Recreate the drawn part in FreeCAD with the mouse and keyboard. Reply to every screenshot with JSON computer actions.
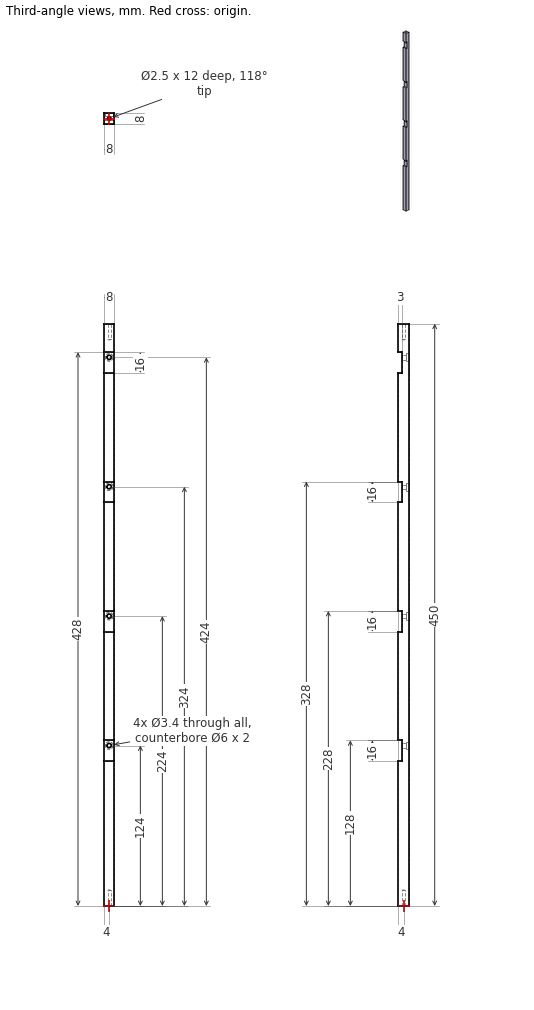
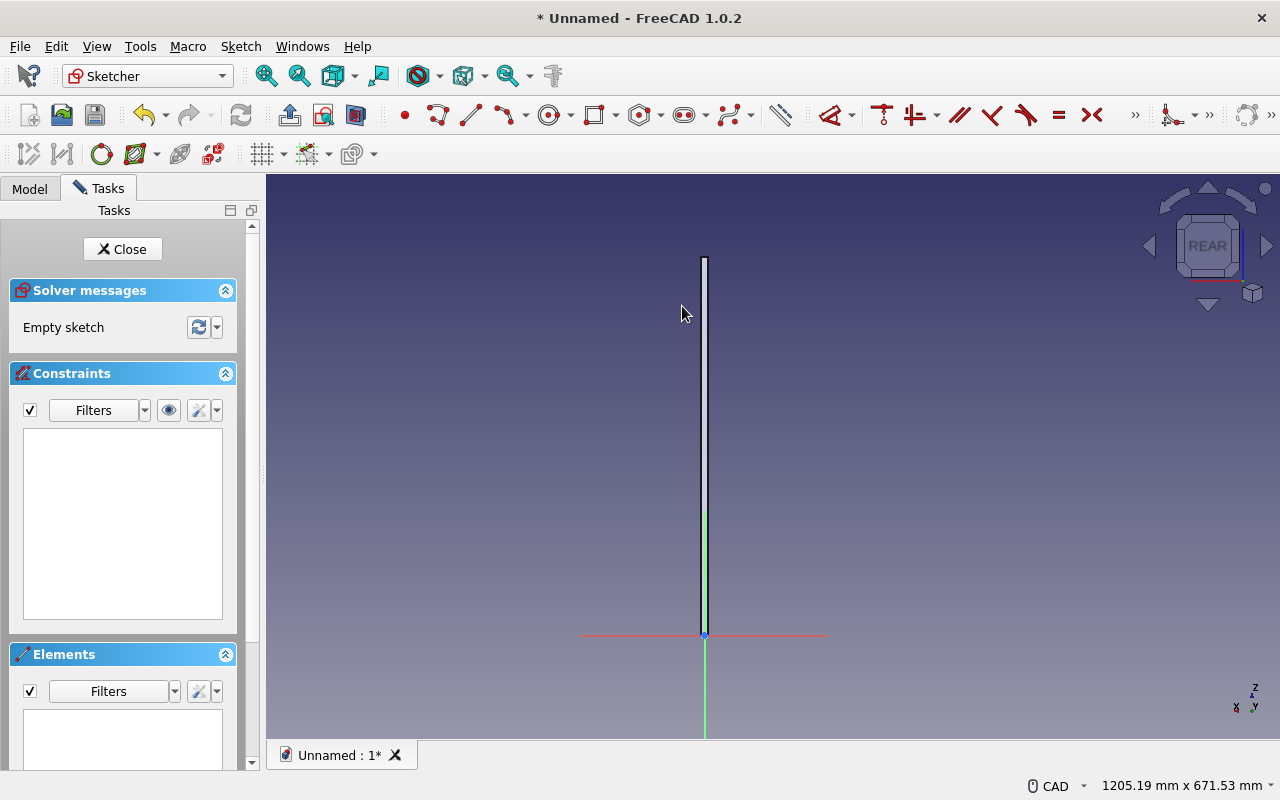
{"action": "key", "text": "g c"}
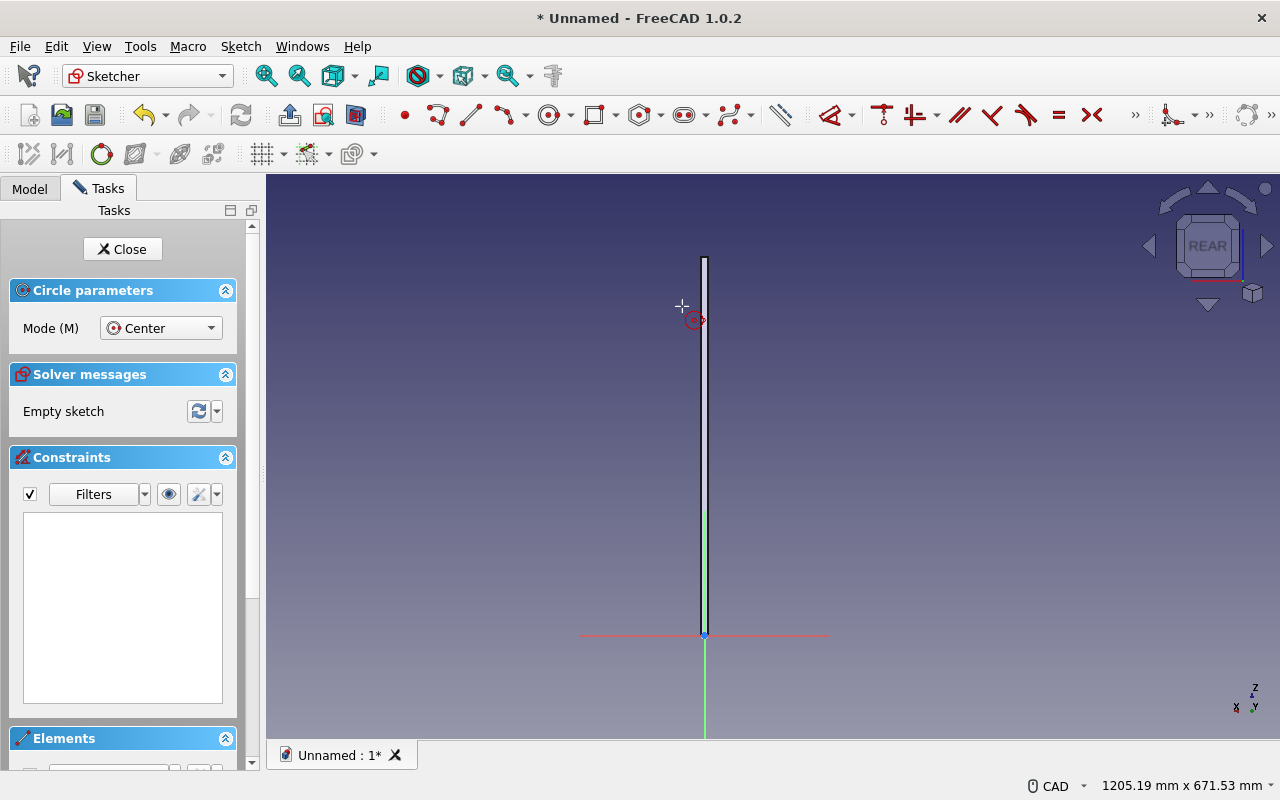
{"action": "scroll", "coordinate": [705, 531], "scroll_direction": "up", "scroll_amount": 14}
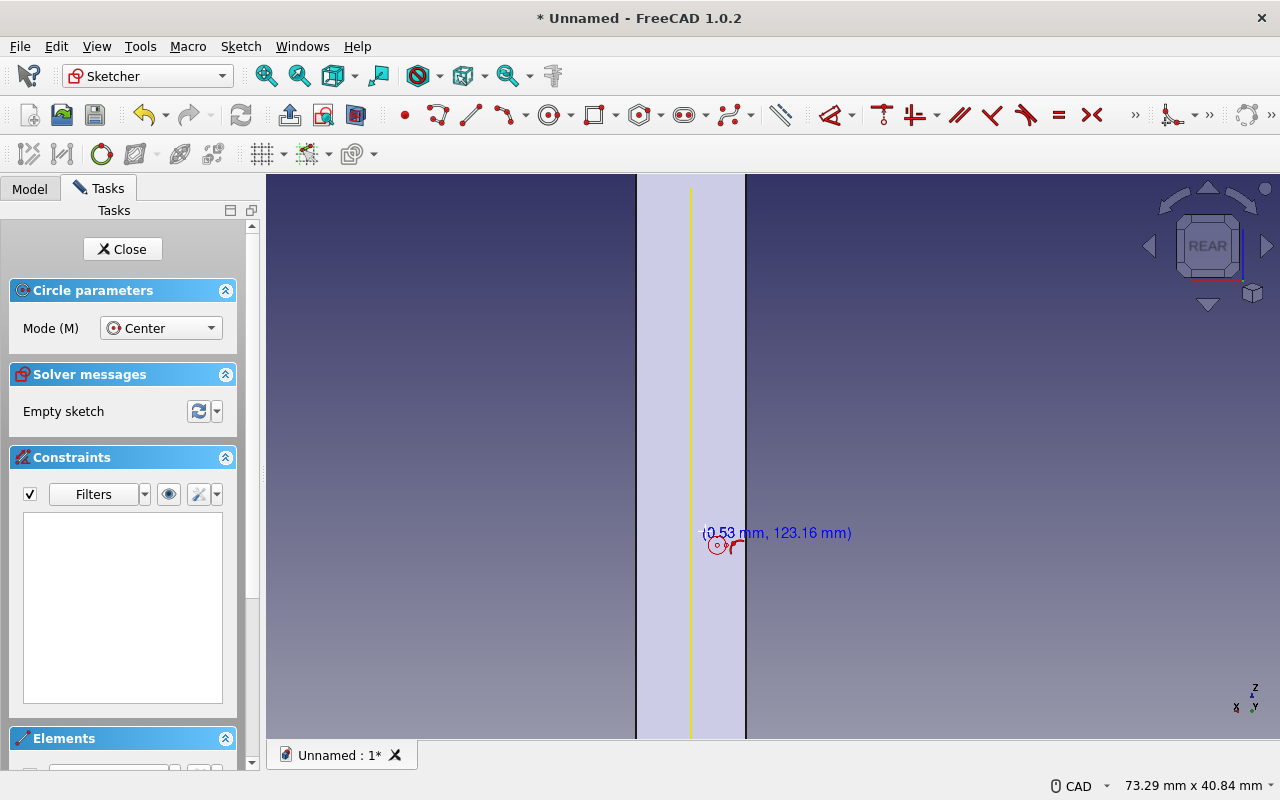
{"action": "scroll", "coordinate": [705, 532], "scroll_direction": "down", "scroll_amount": 14}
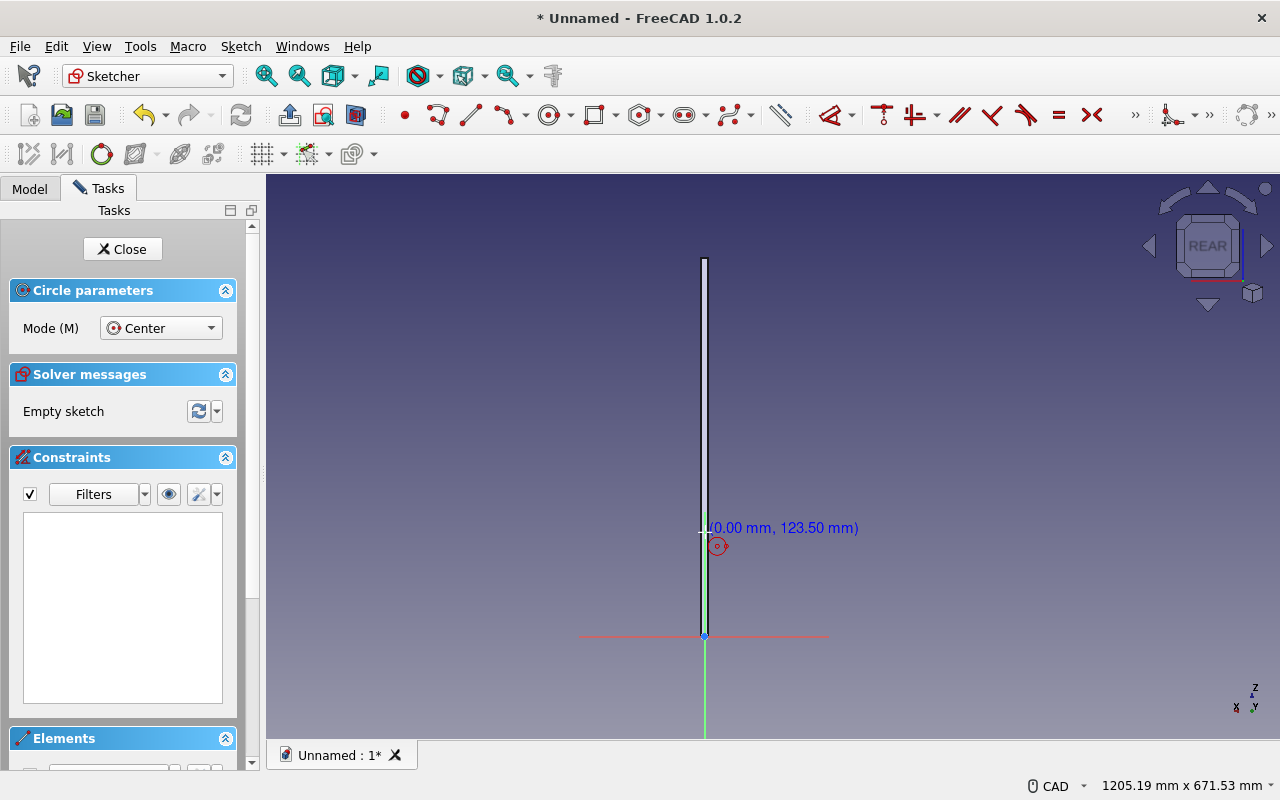
{"action": "left_click", "coordinate": [705, 532]}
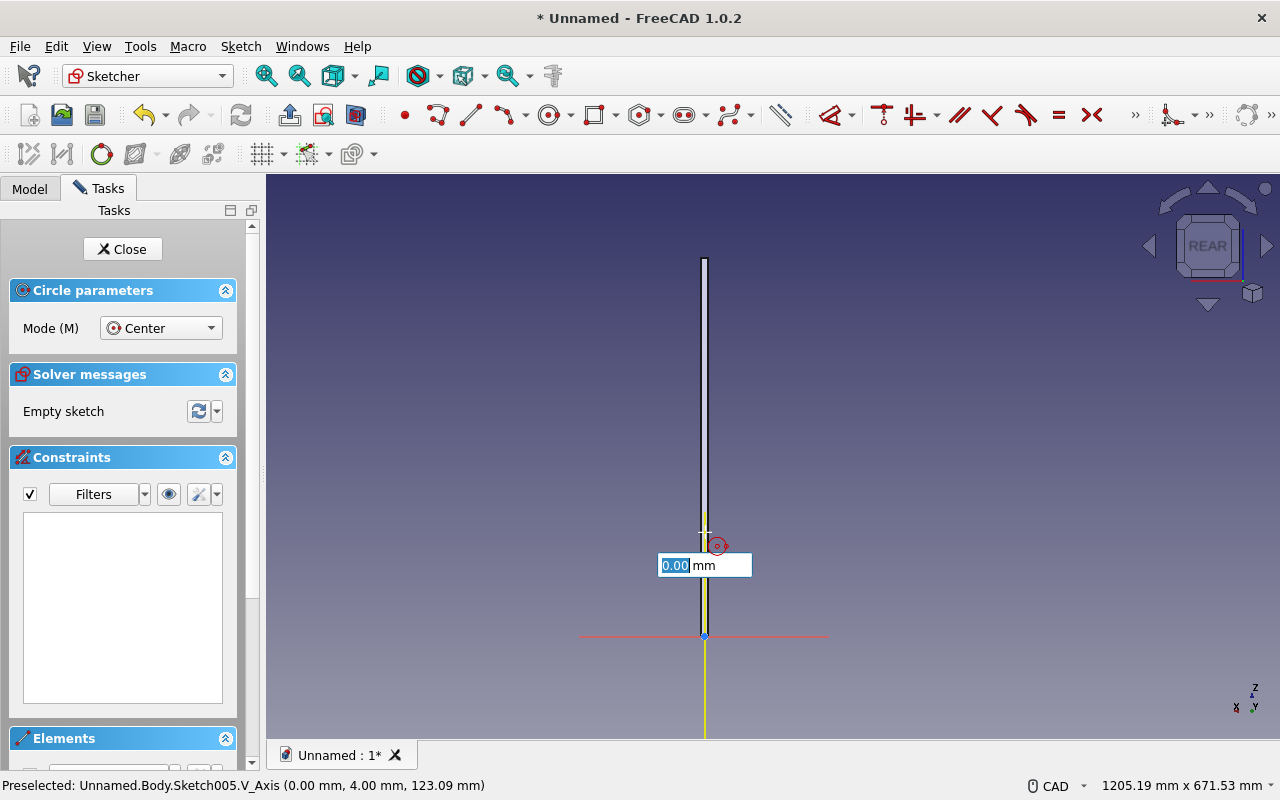
{"action": "scroll", "coordinate": [706, 532], "scroll_direction": "up", "scroll_amount": 13}
{"action": "mouse_move", "coordinate": [699, 521]}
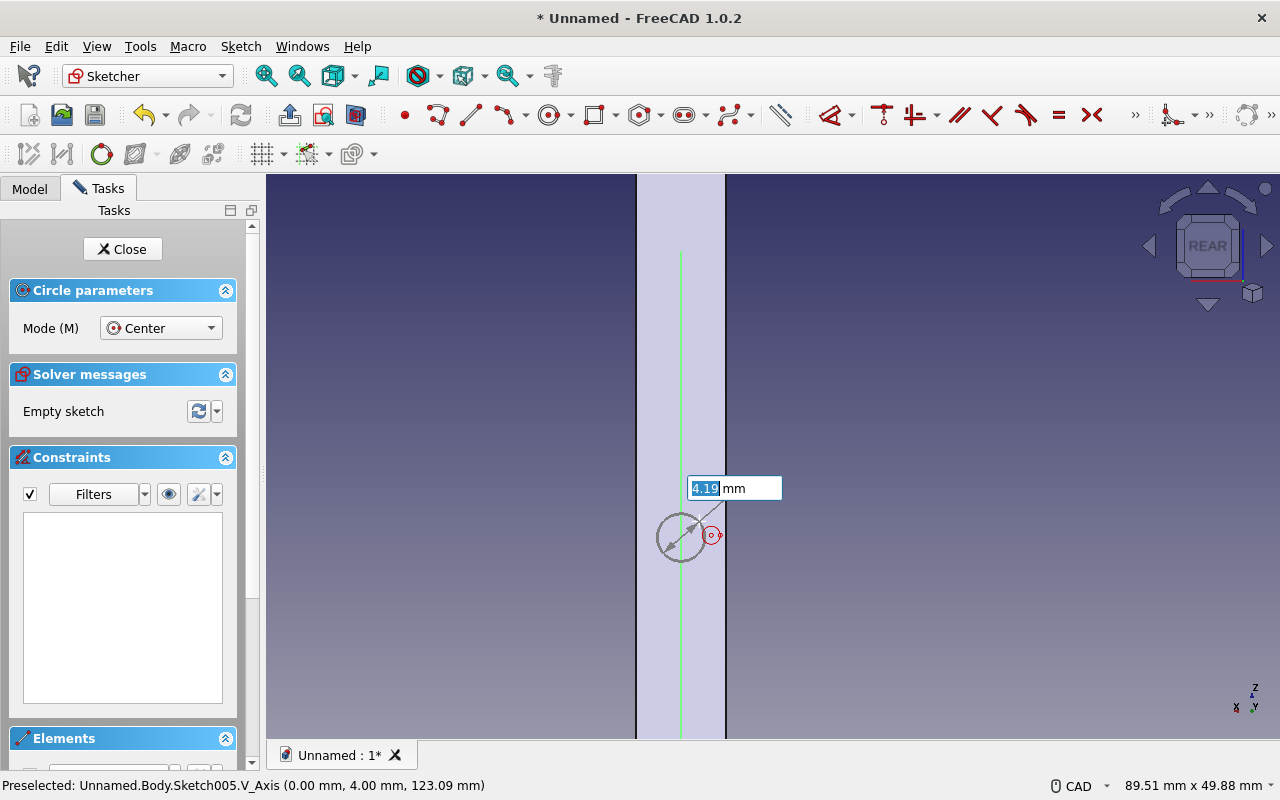
{"action": "type", "text": "3.4"}
{"action": "key", "text": "Return"}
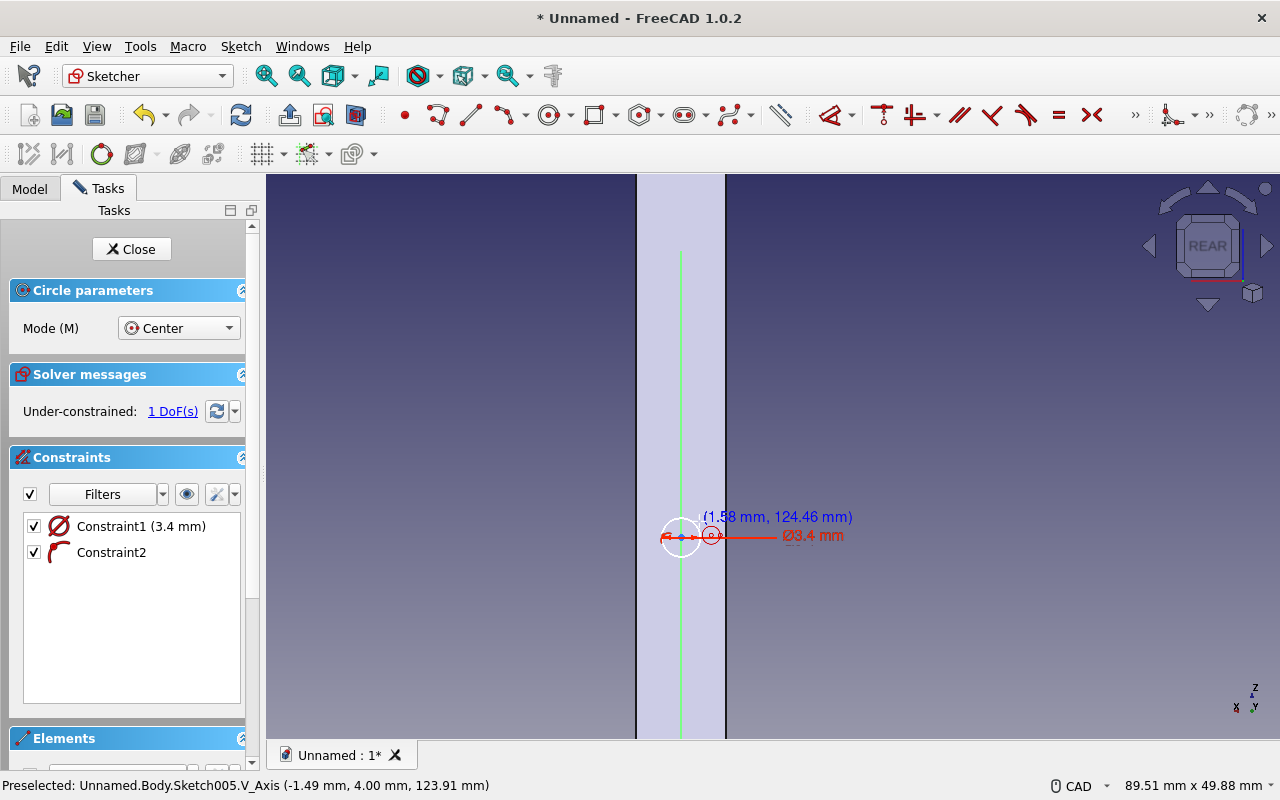
{"action": "scroll", "coordinate": [706, 532], "scroll_direction": "down", "scroll_amount": 13}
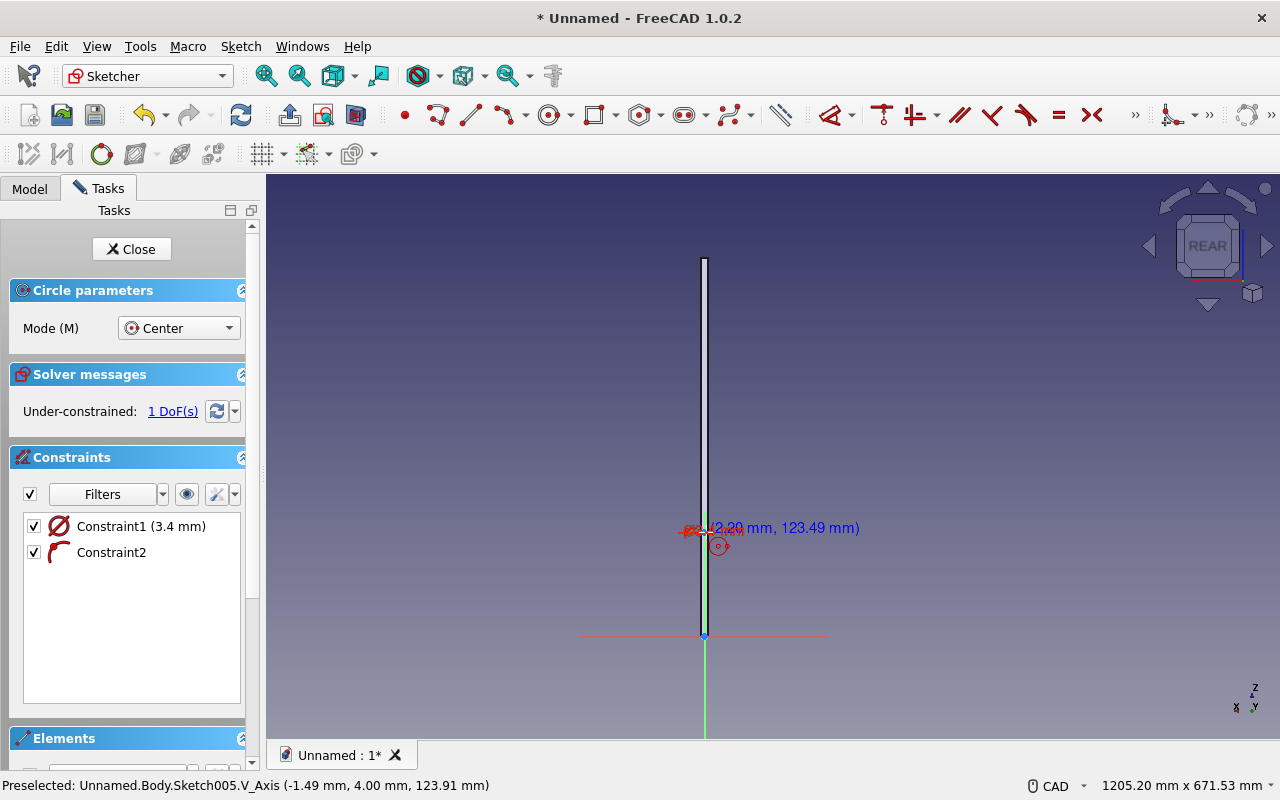
{"action": "scroll", "coordinate": [705, 448], "scroll_direction": "up", "scroll_amount": 14}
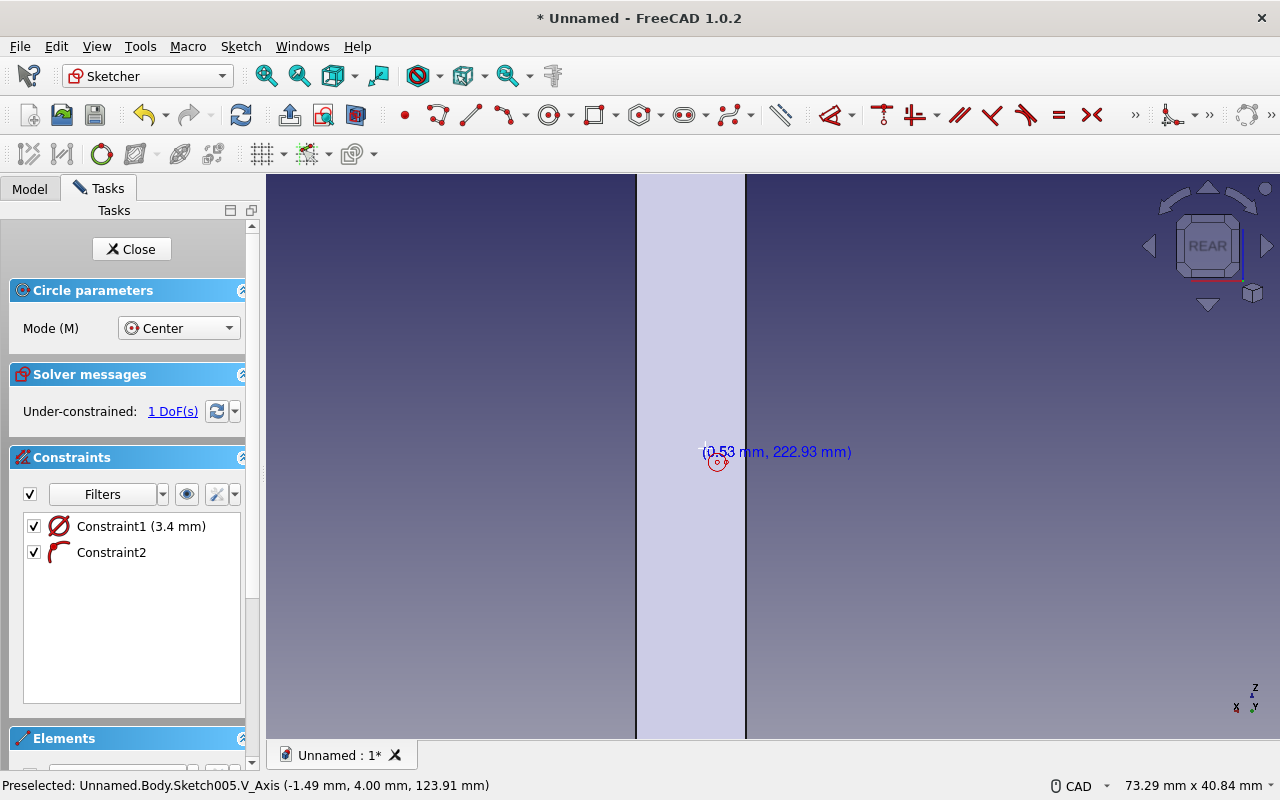
{"action": "scroll", "coordinate": [705, 447], "scroll_direction": "down", "scroll_amount": 14}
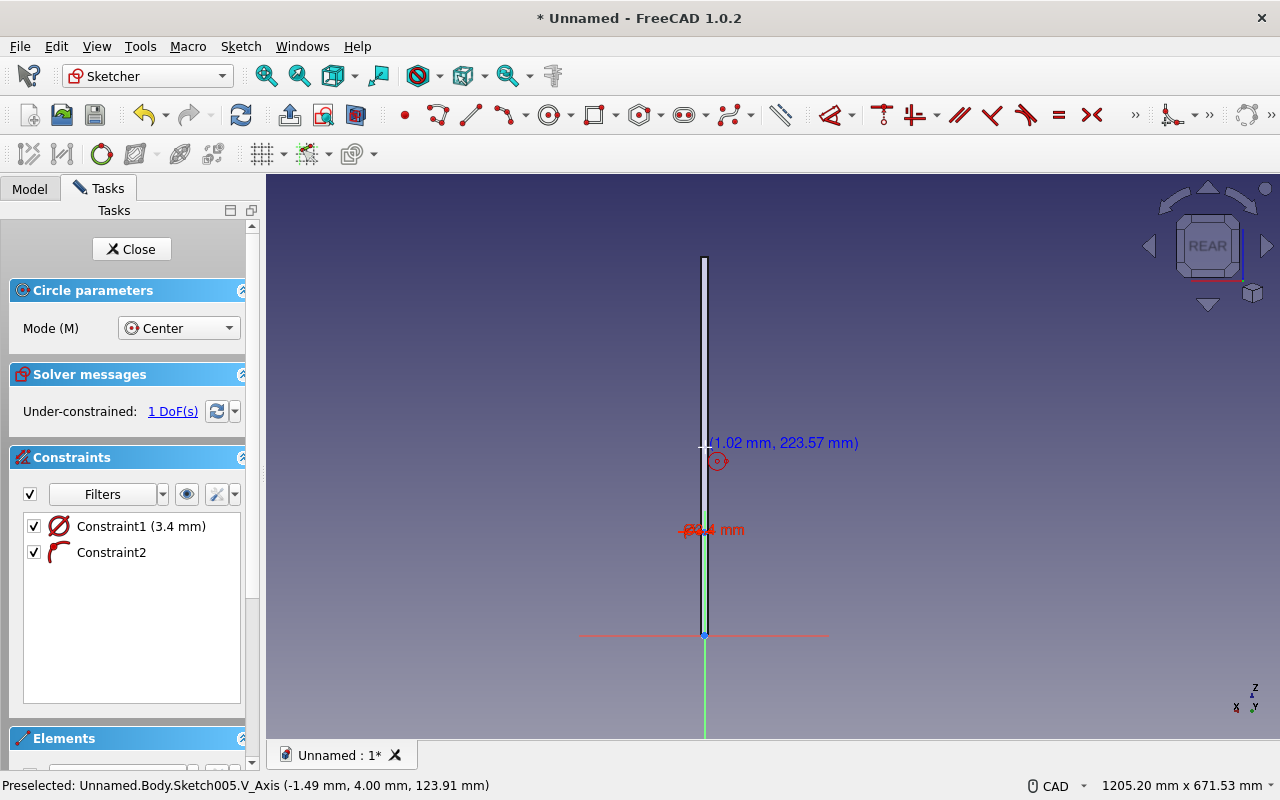
{"action": "left_click", "coordinate": [705, 447]}